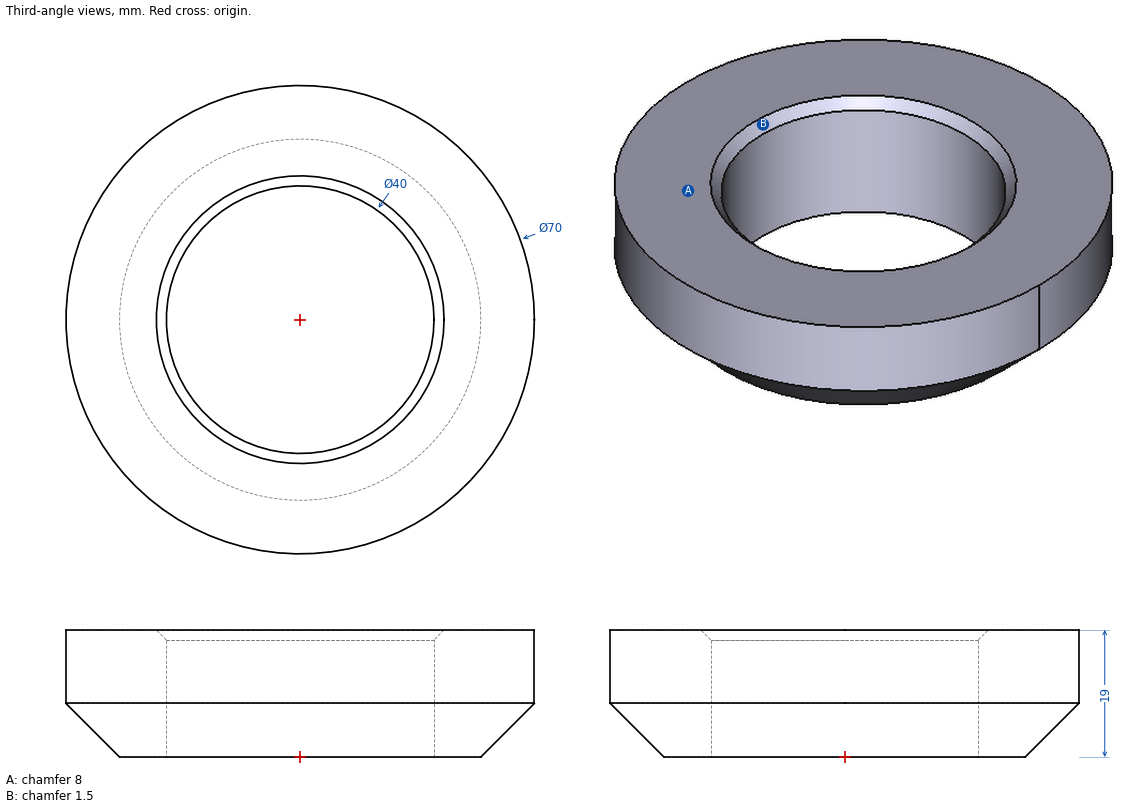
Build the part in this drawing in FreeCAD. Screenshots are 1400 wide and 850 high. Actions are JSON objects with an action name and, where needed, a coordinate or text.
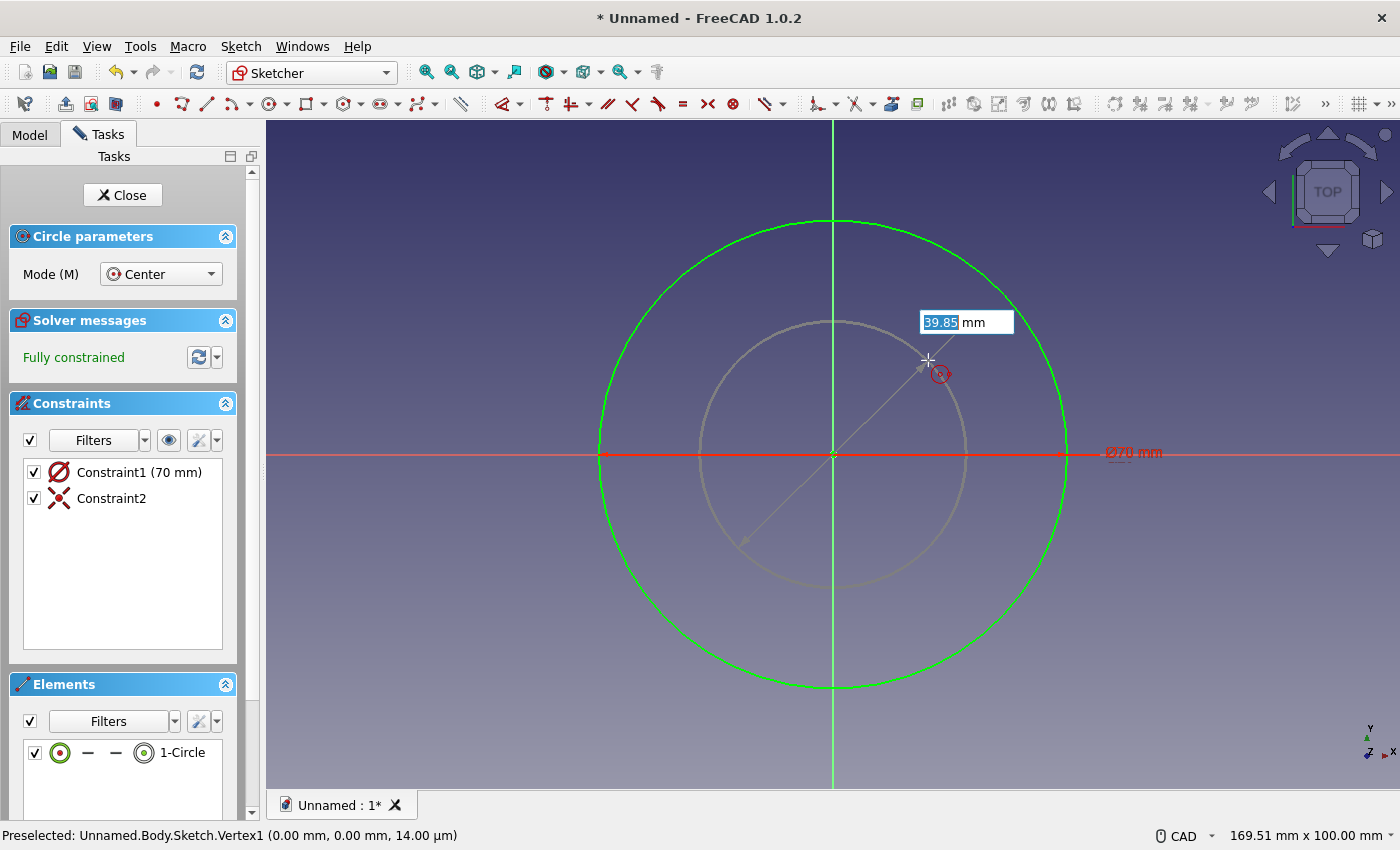
{"action": "type", "text": "40"}
{"action": "key", "text": "Return"}
{"action": "key", "text": "Escape"}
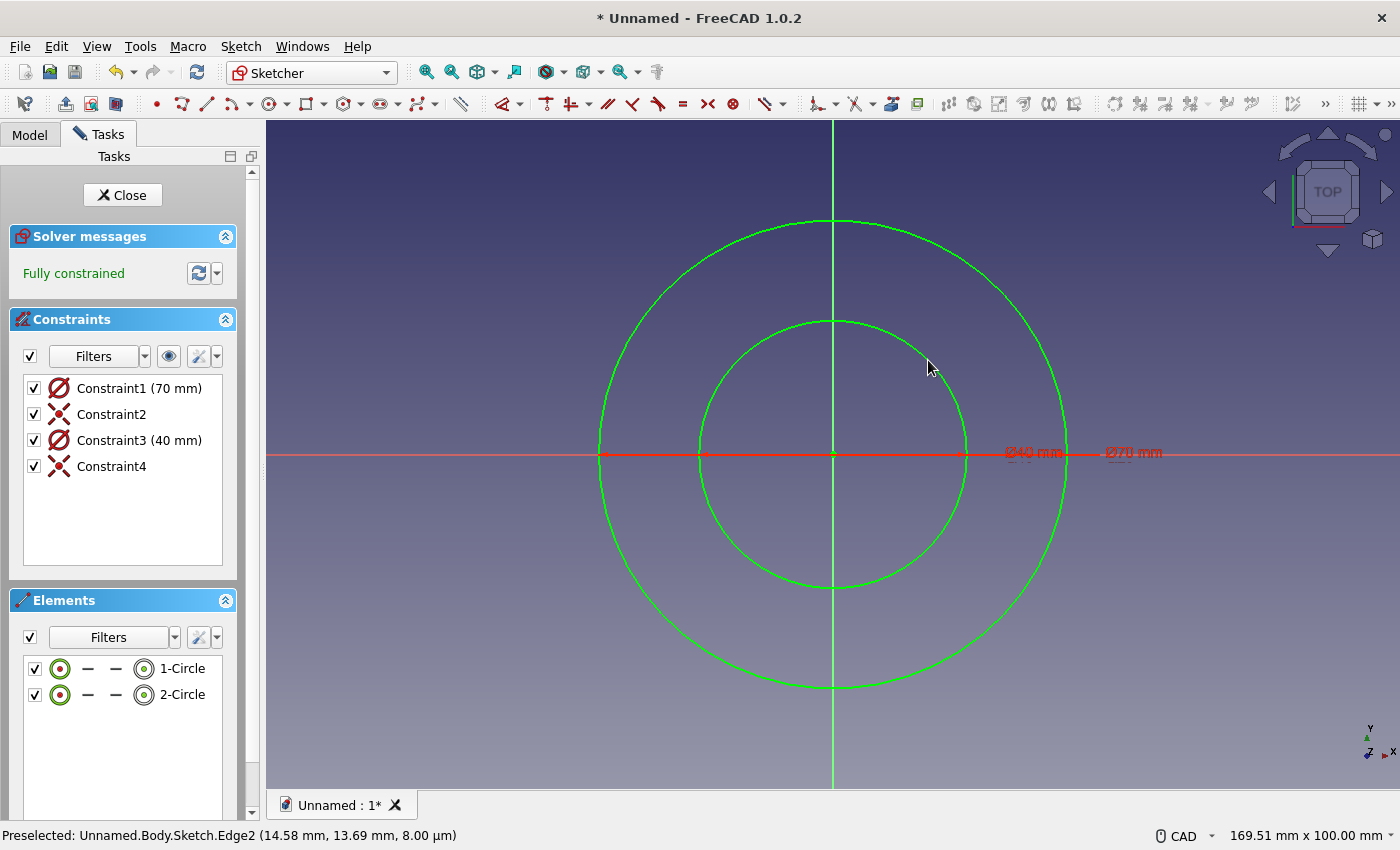
{"action": "left_click", "coordinate": [123, 195]}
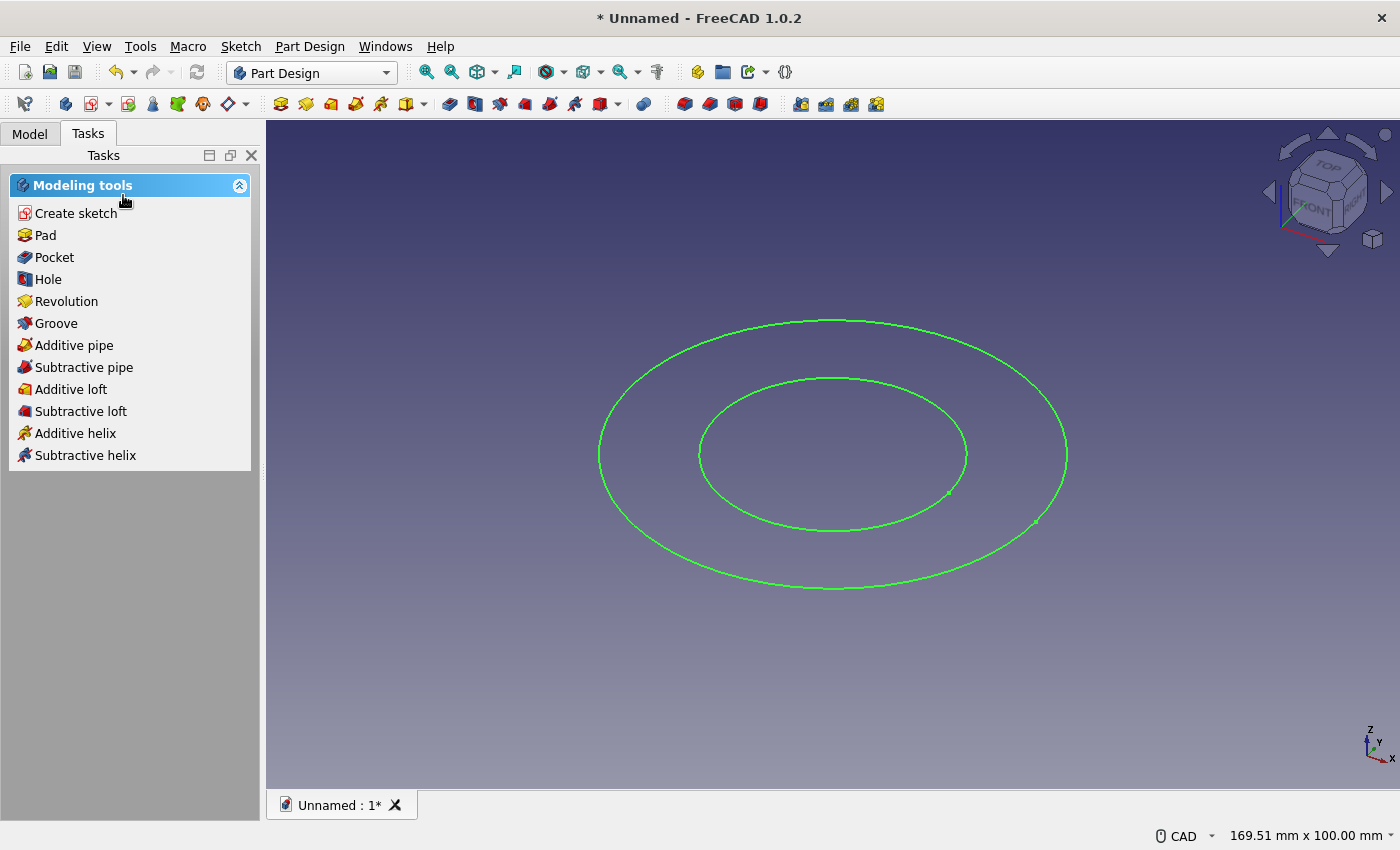
{"action": "left_click", "coordinate": [281, 104]}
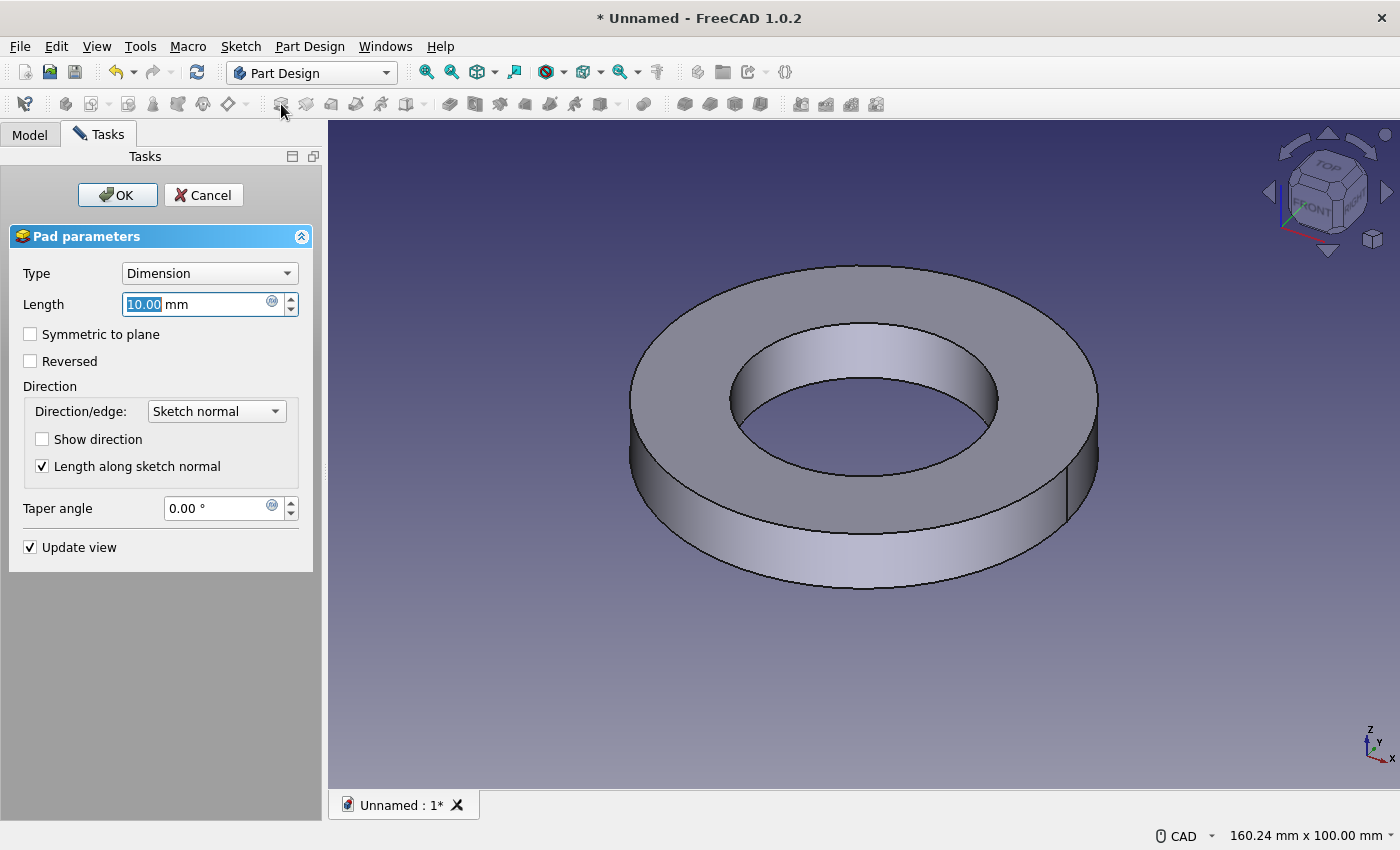
{"action": "type", "text": "19"}
{"action": "key", "text": "Tab"}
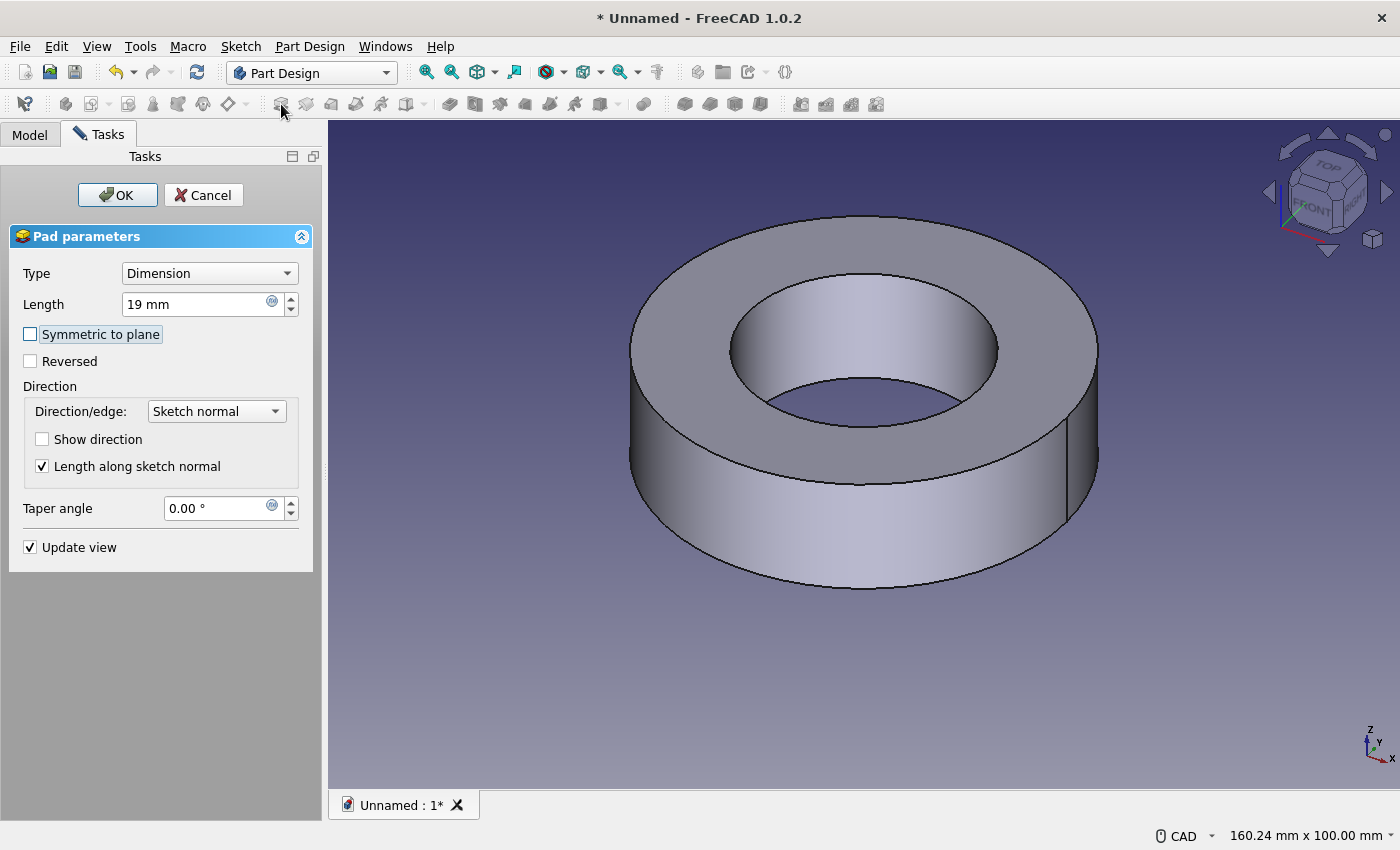
{"action": "left_click", "coordinate": [118, 195]}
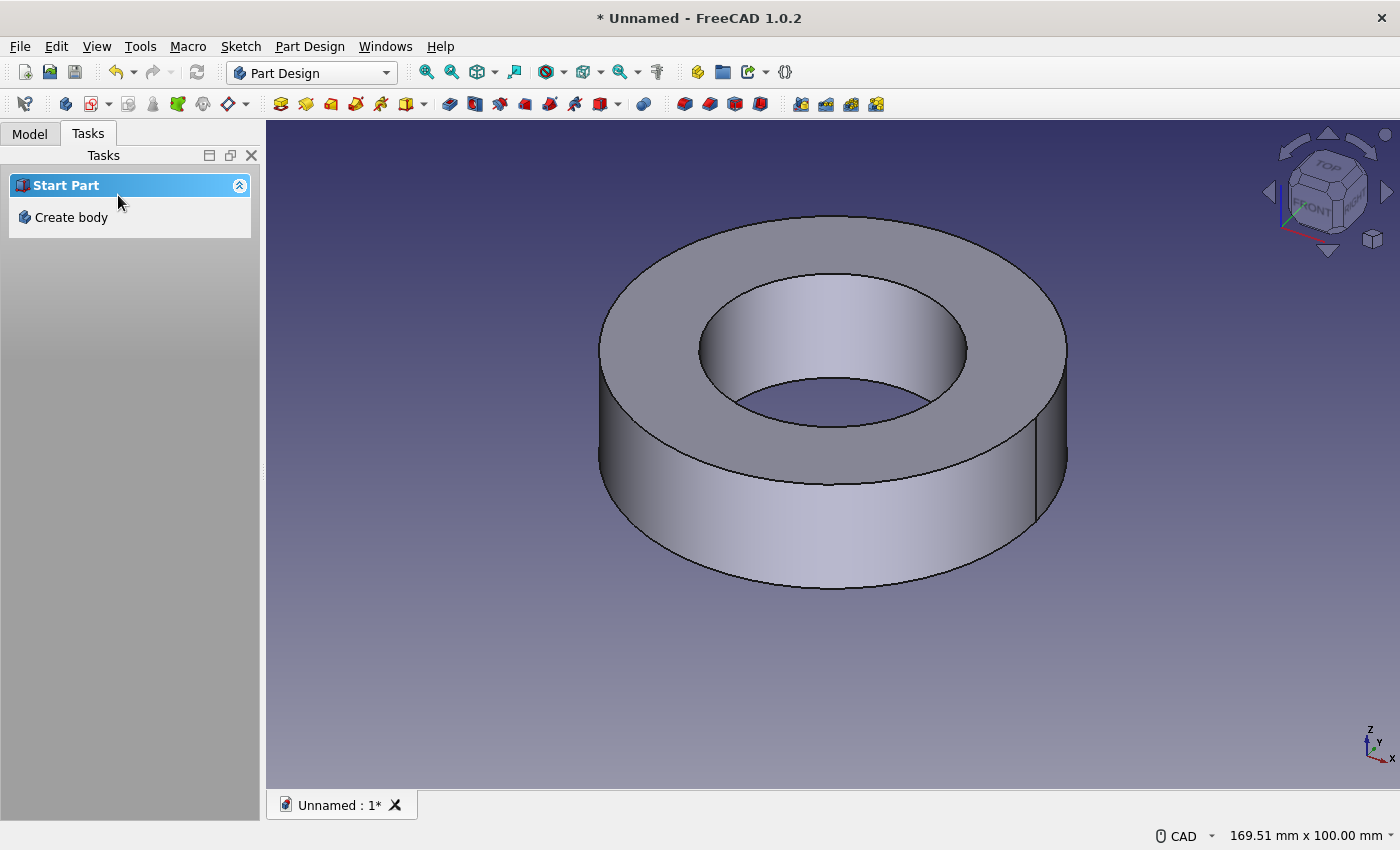
{"action": "key", "text": "0"}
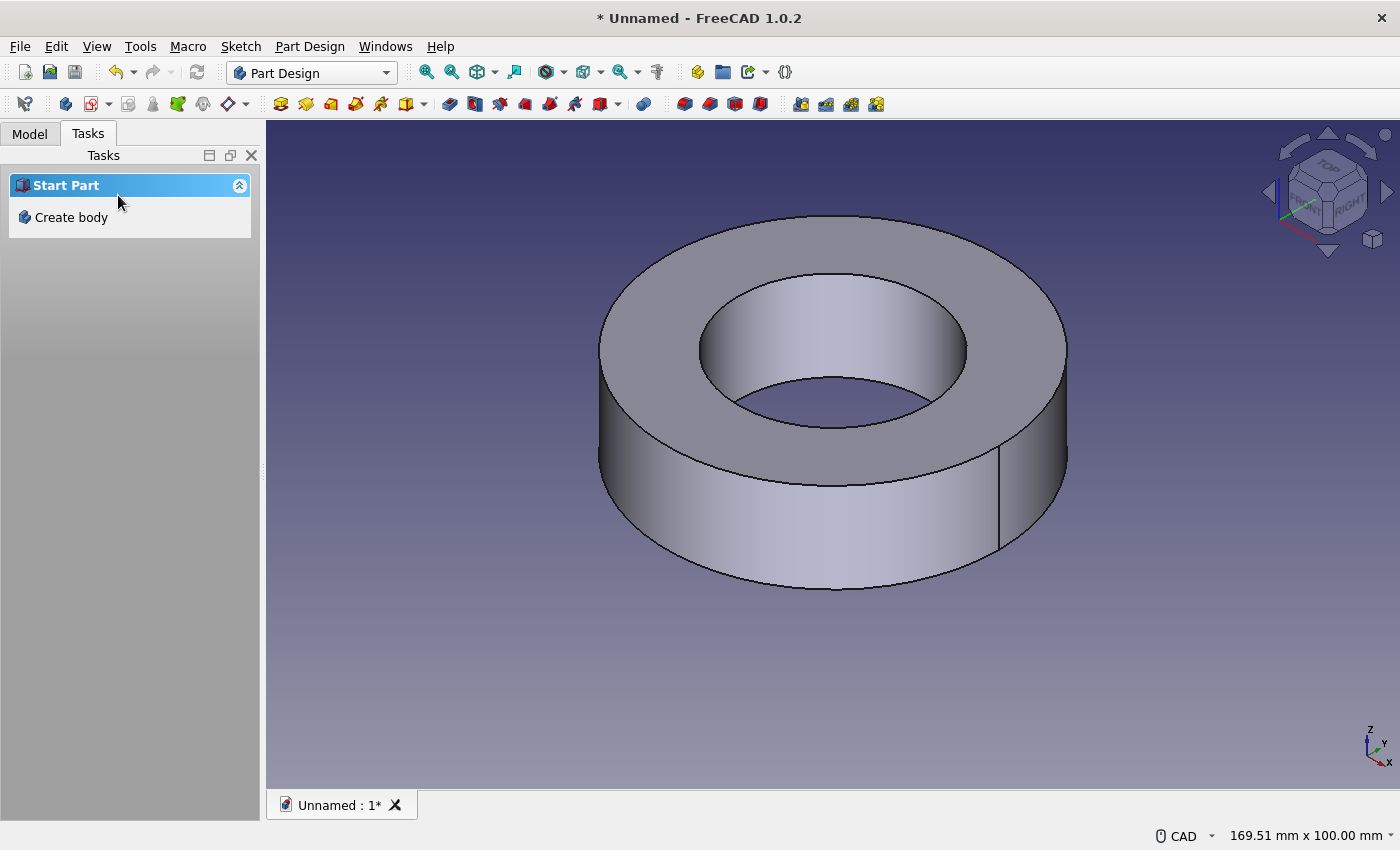
{"action": "key", "text": "2"}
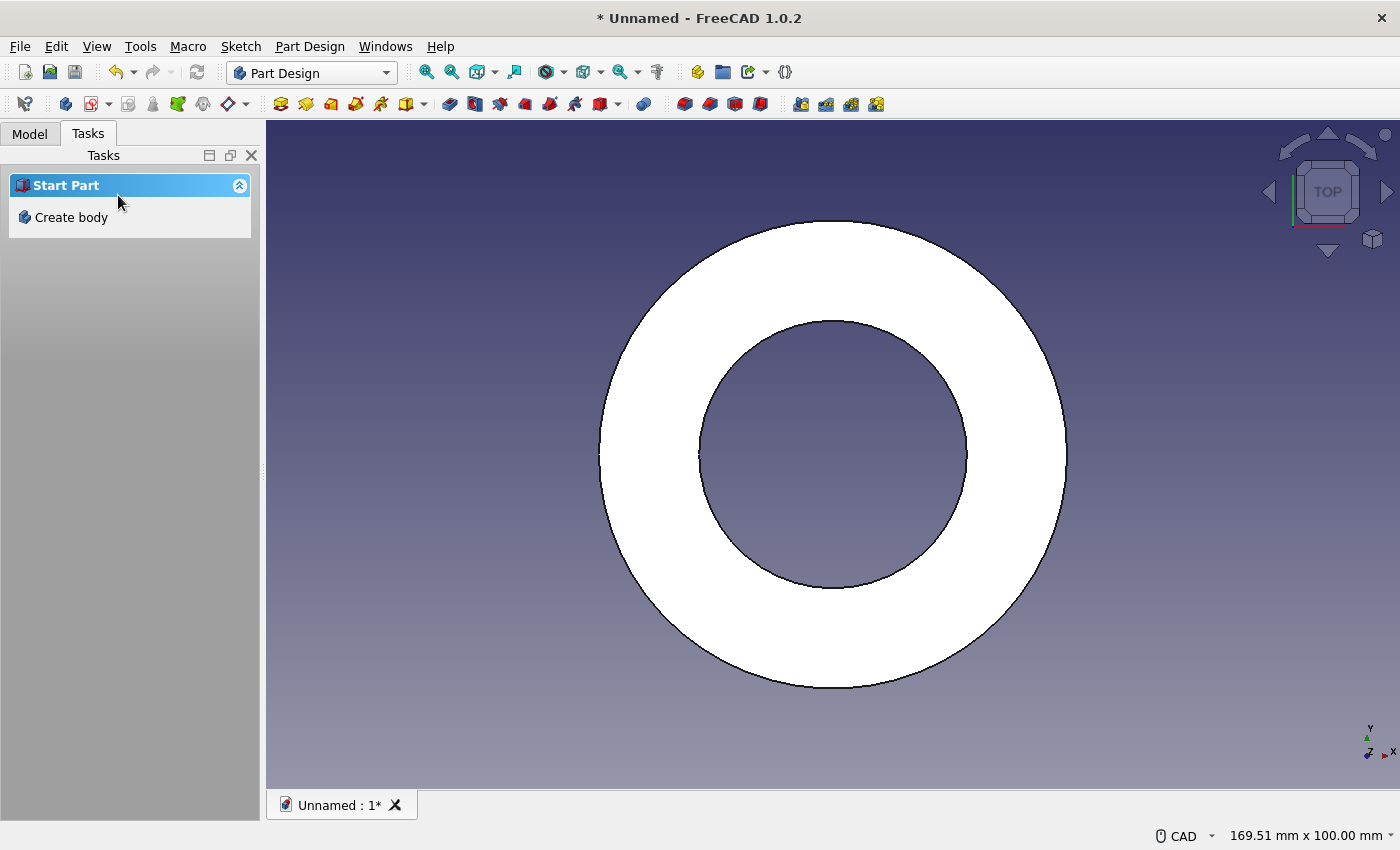
{"action": "key", "text": "1"}